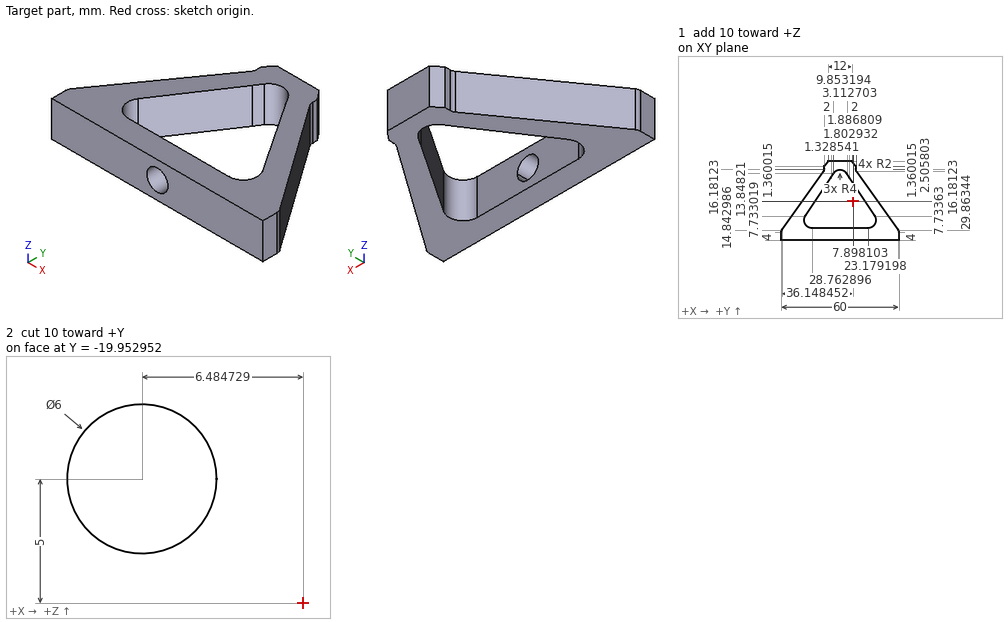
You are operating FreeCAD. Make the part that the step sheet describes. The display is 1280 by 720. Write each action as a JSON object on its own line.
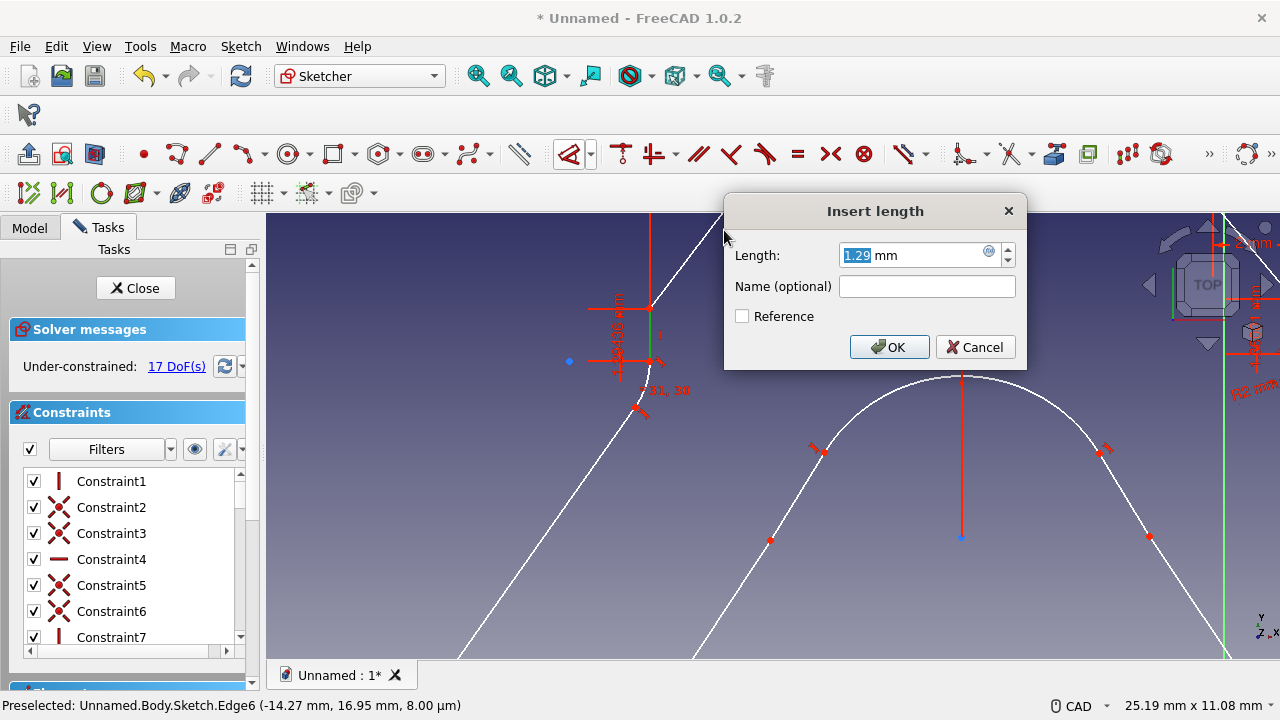
{"action": "type", "text": "1.360015"}
{"action": "key", "text": "Return"}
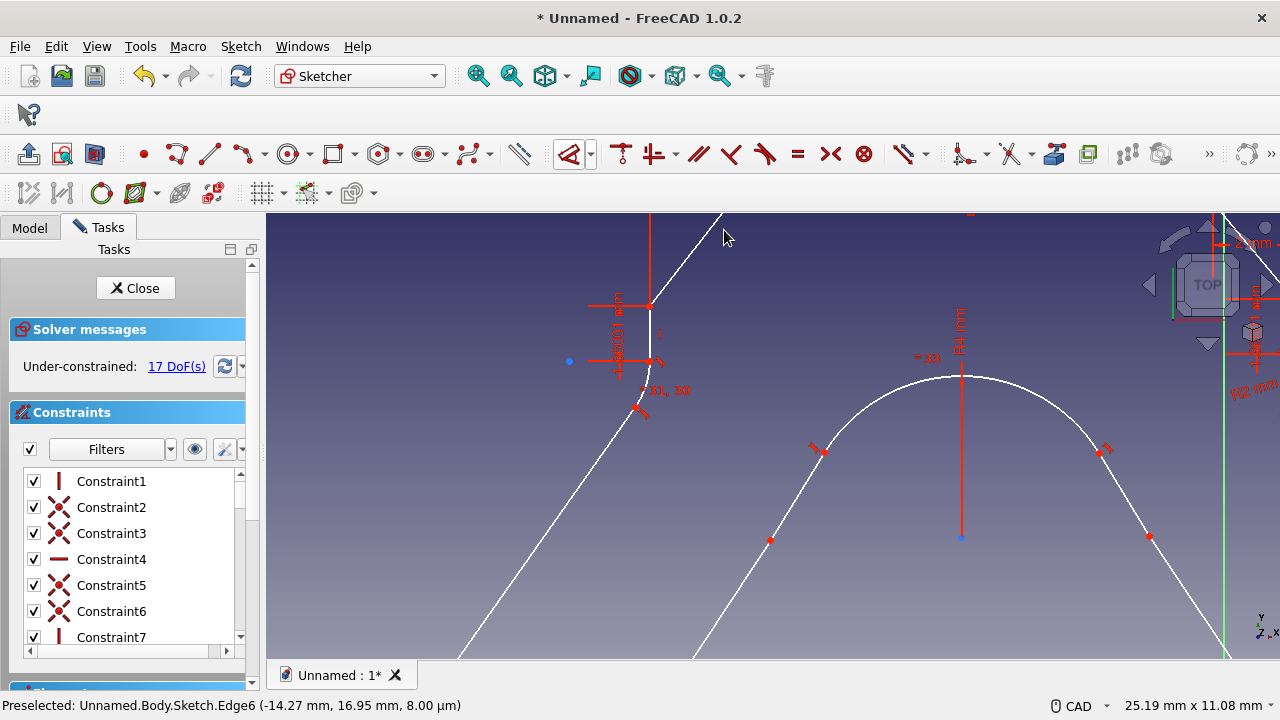
{"action": "scroll", "coordinate": [653, 323], "scroll_direction": "down", "scroll_amount": 9}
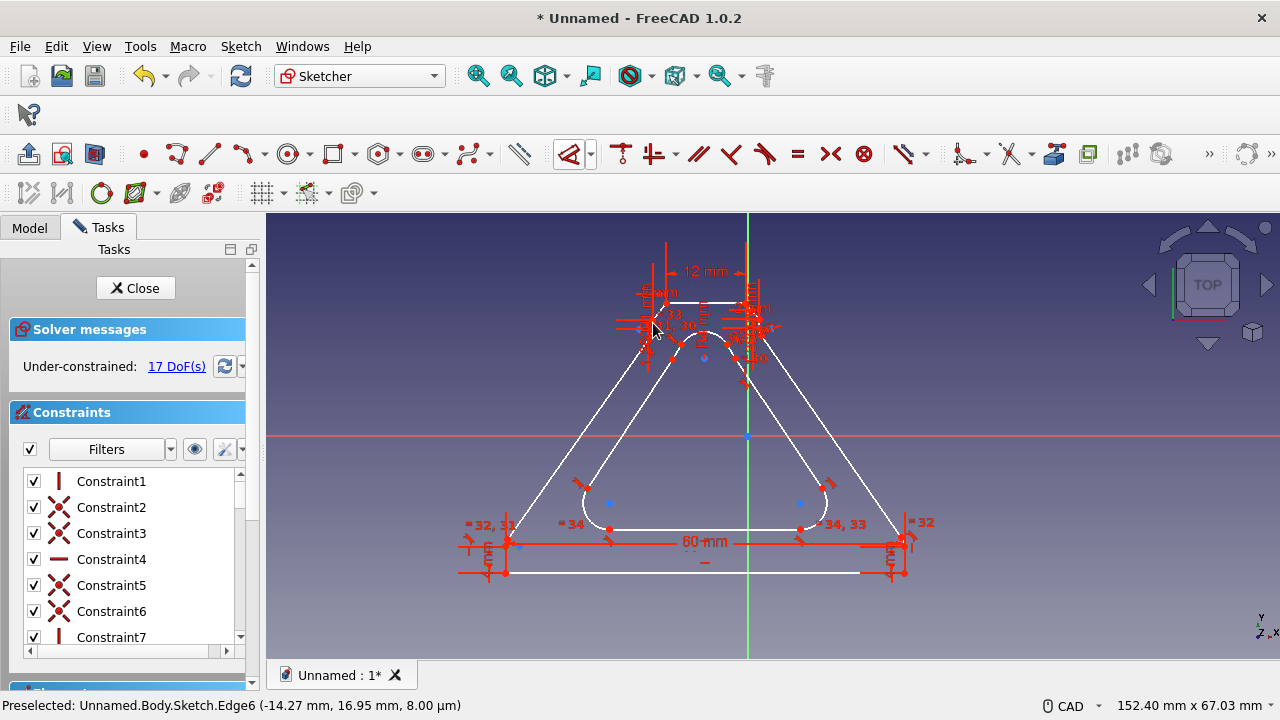
{"action": "left_click", "coordinate": [822, 488]}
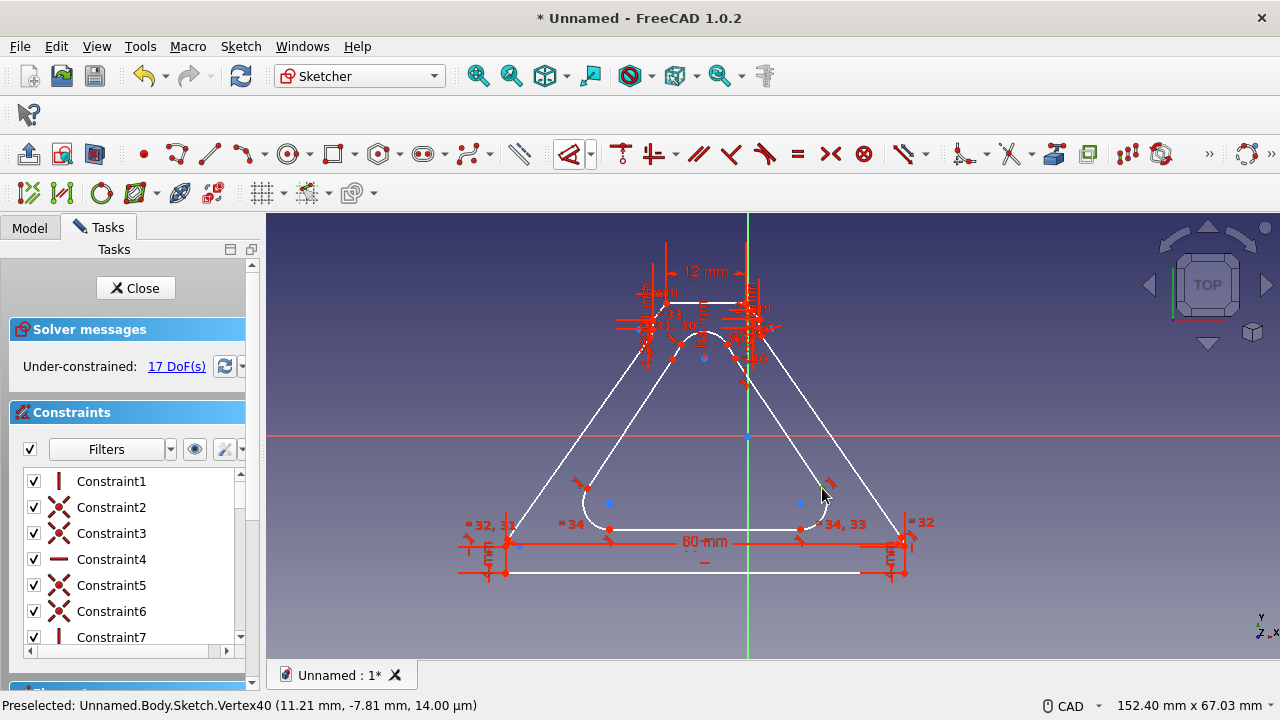
{"action": "left_click", "coordinate": [590, 154]}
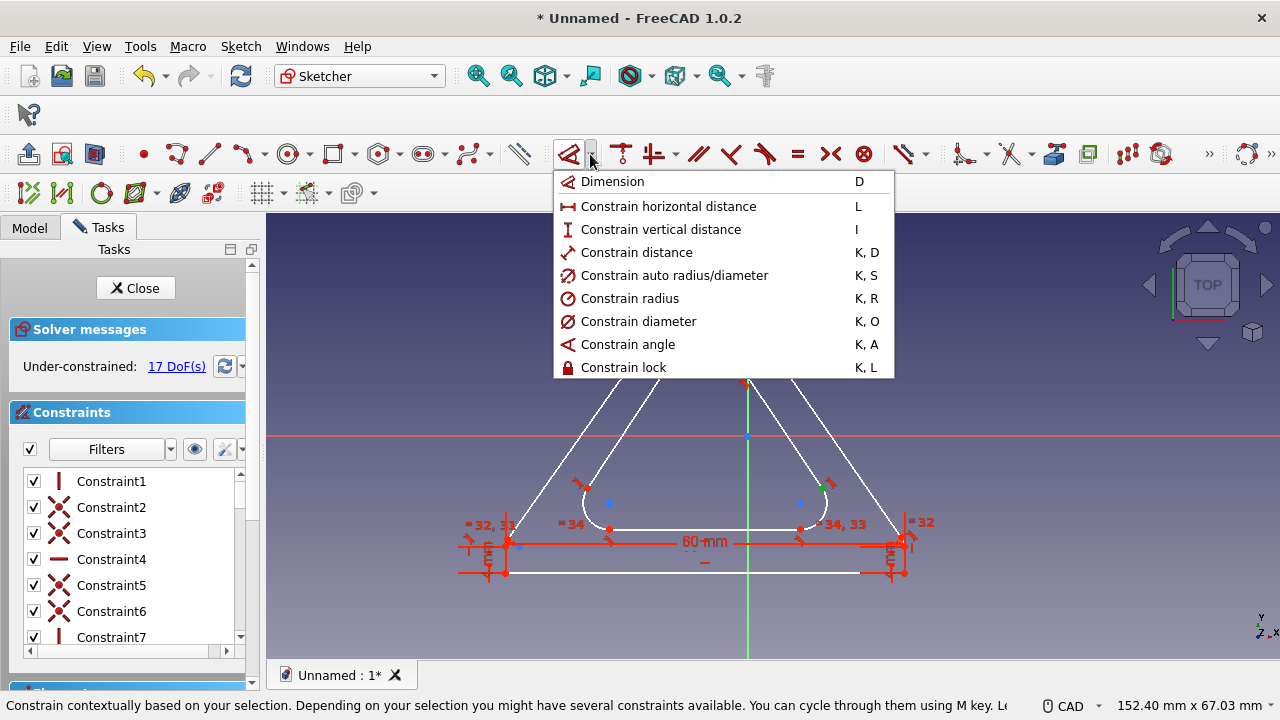
{"action": "left_click", "coordinate": [724, 230]}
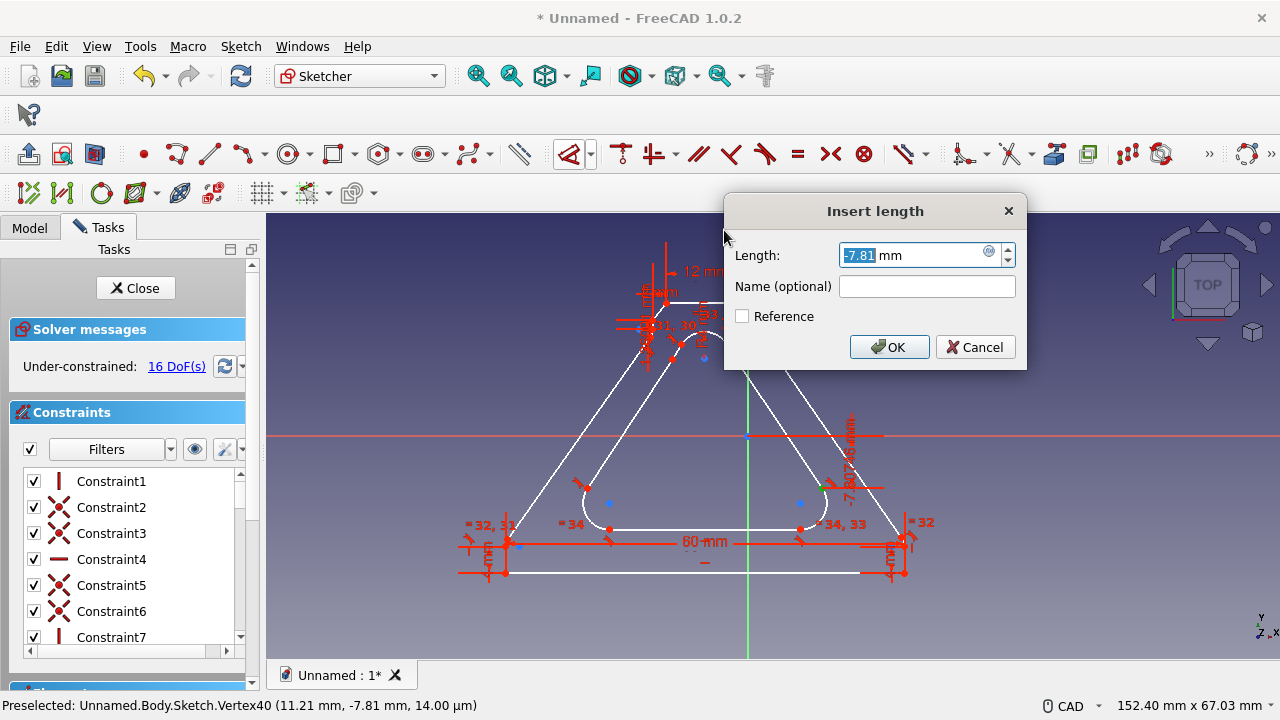
{"action": "type", "text": "-7.73363"}
{"action": "key", "text": "Return"}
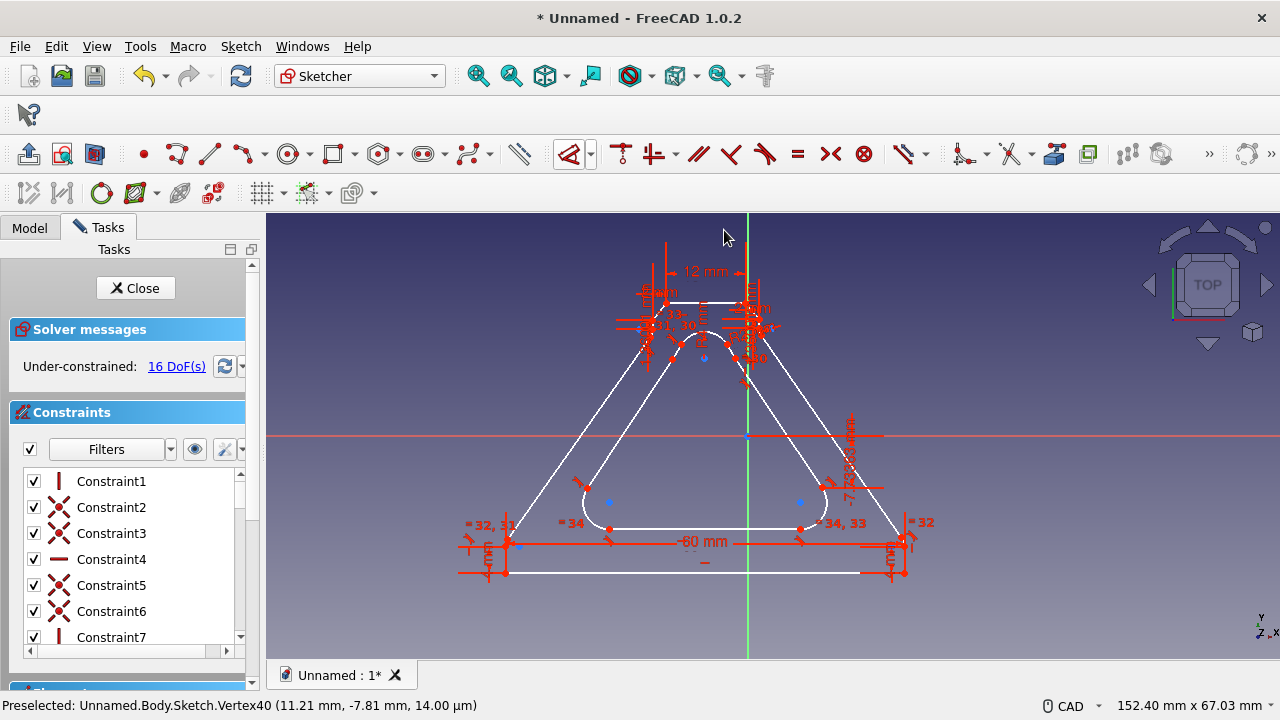
{"action": "left_click", "coordinate": [667, 529]}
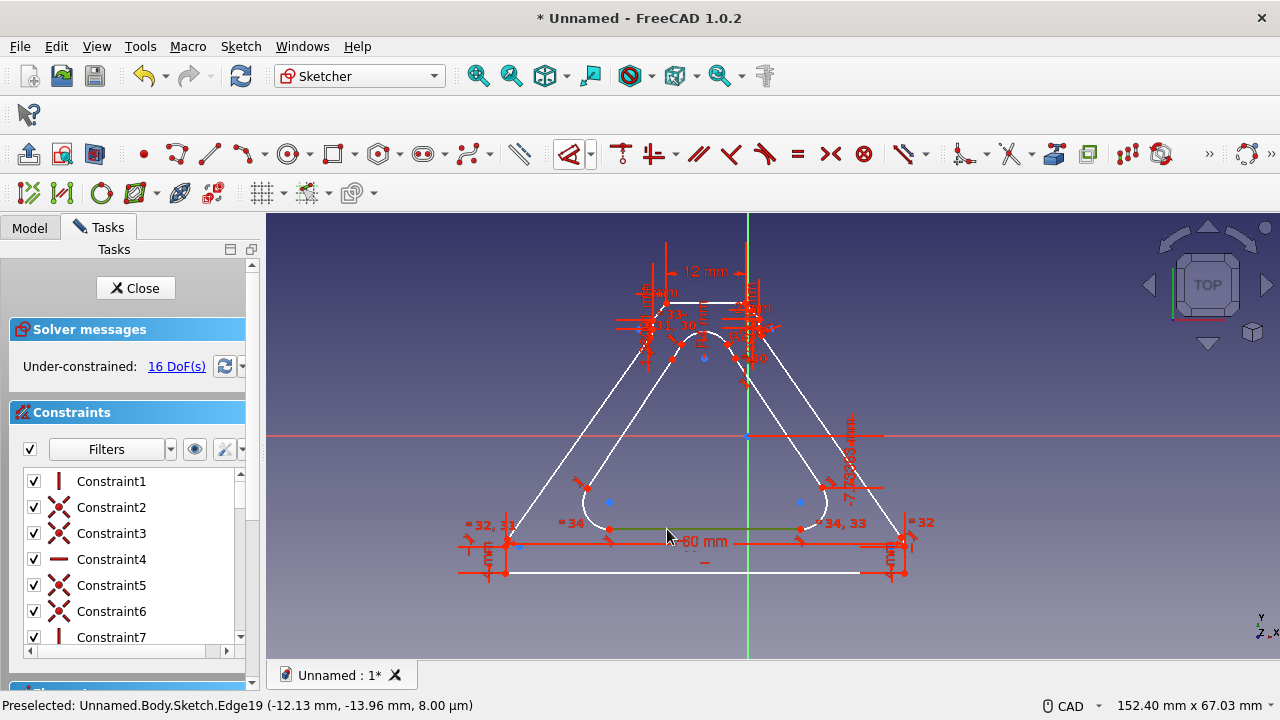
{"action": "key", "text": "l"}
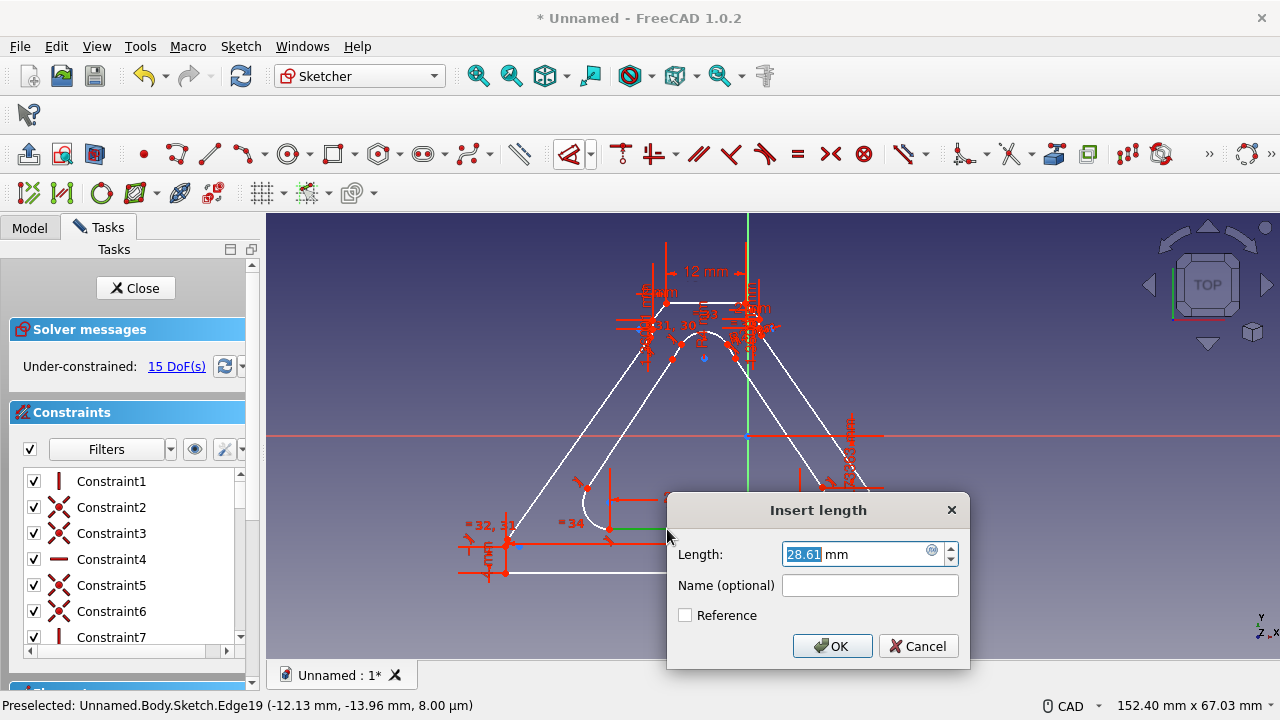
{"action": "type", "text": "28.762896"}
{"action": "key", "text": "Return"}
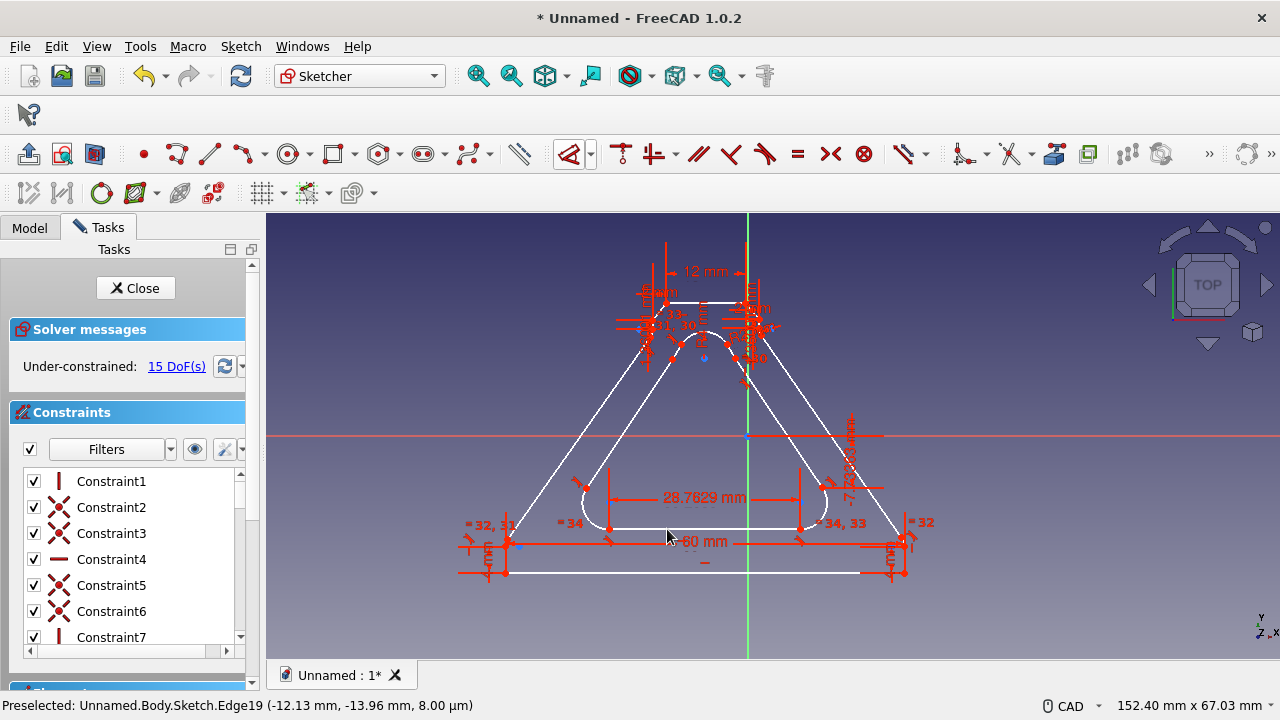
{"action": "scroll", "coordinate": [762, 336], "scroll_direction": "up", "scroll_amount": 6}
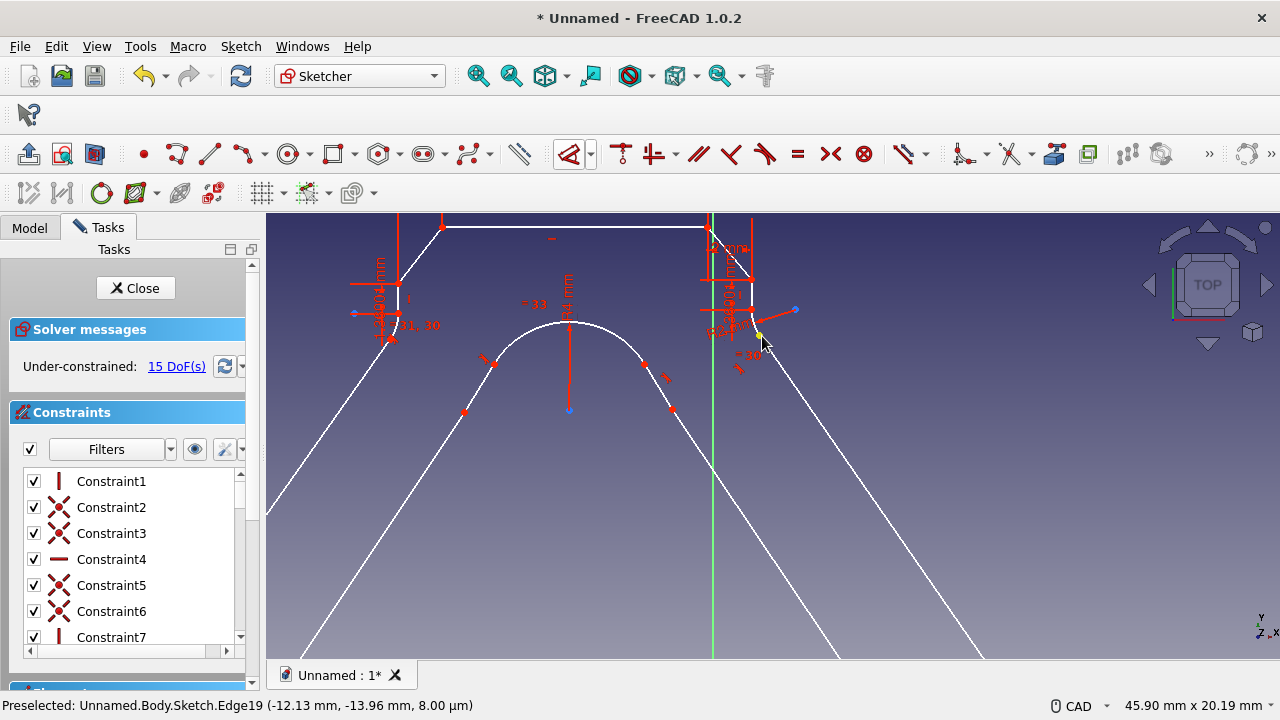
{"action": "left_click", "coordinate": [760, 335]}